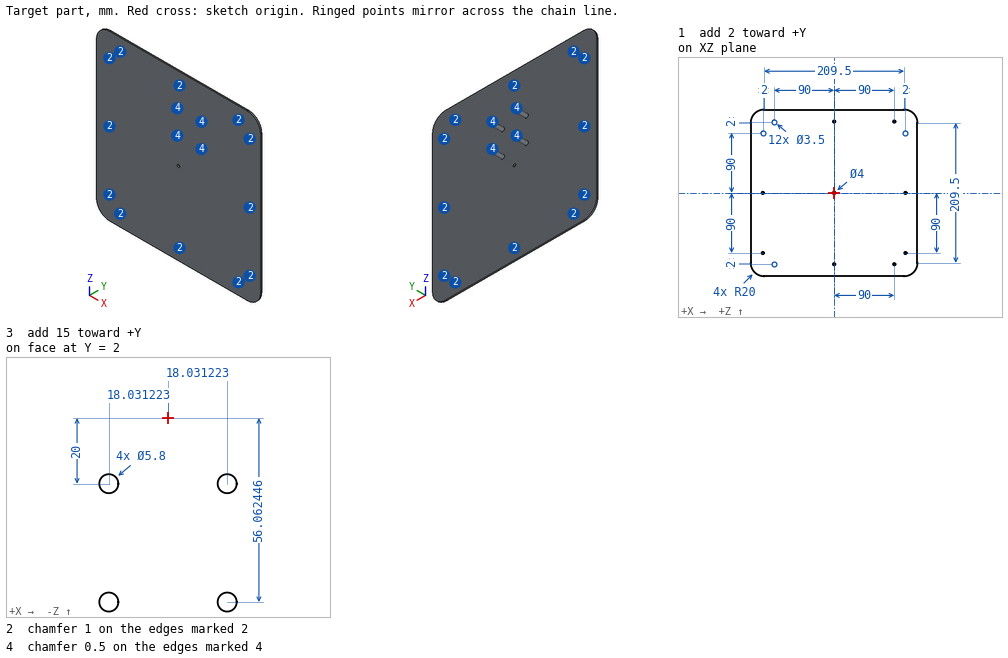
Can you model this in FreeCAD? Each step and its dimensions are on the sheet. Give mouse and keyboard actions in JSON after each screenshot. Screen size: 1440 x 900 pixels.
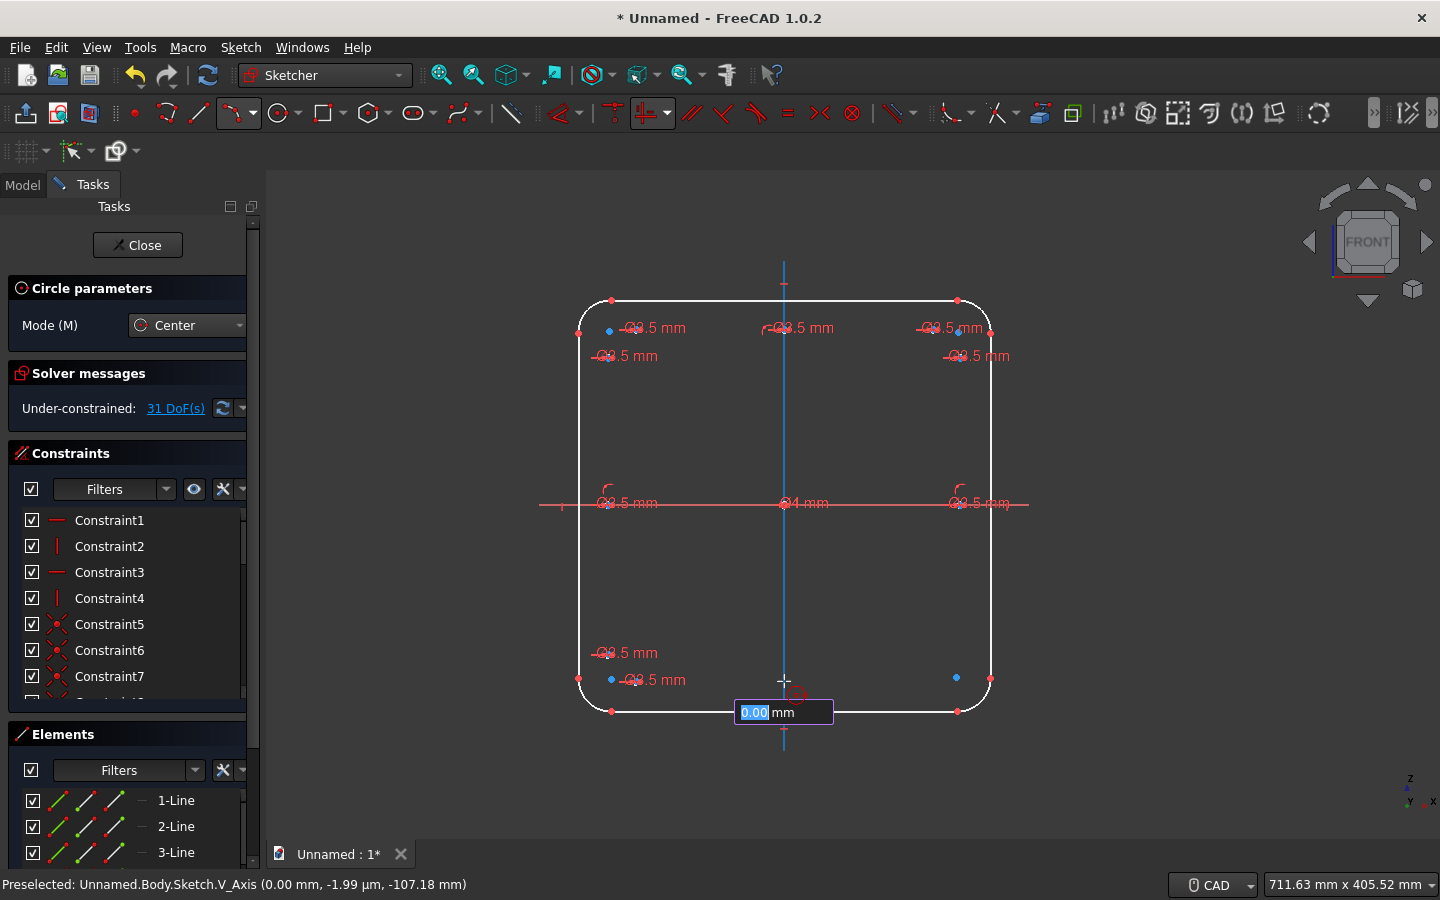
{"action": "scroll", "coordinate": [787, 680], "scroll_direction": "up", "scroll_amount": 9}
{"action": "mouse_move", "coordinate": [786, 678]}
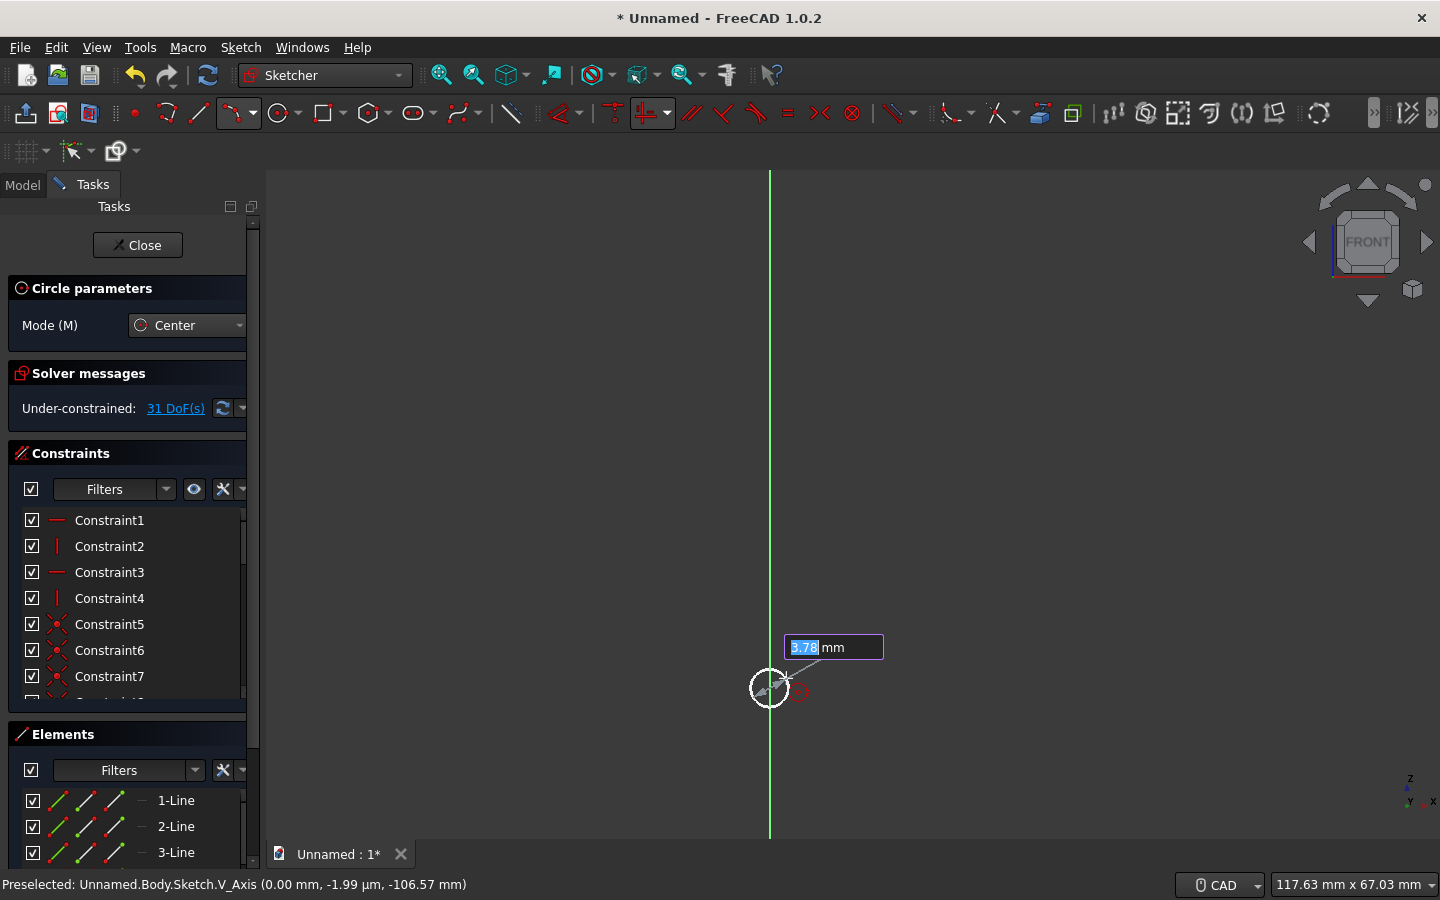
{"action": "type", "text": "3.5"}
{"action": "key", "text": "Return"}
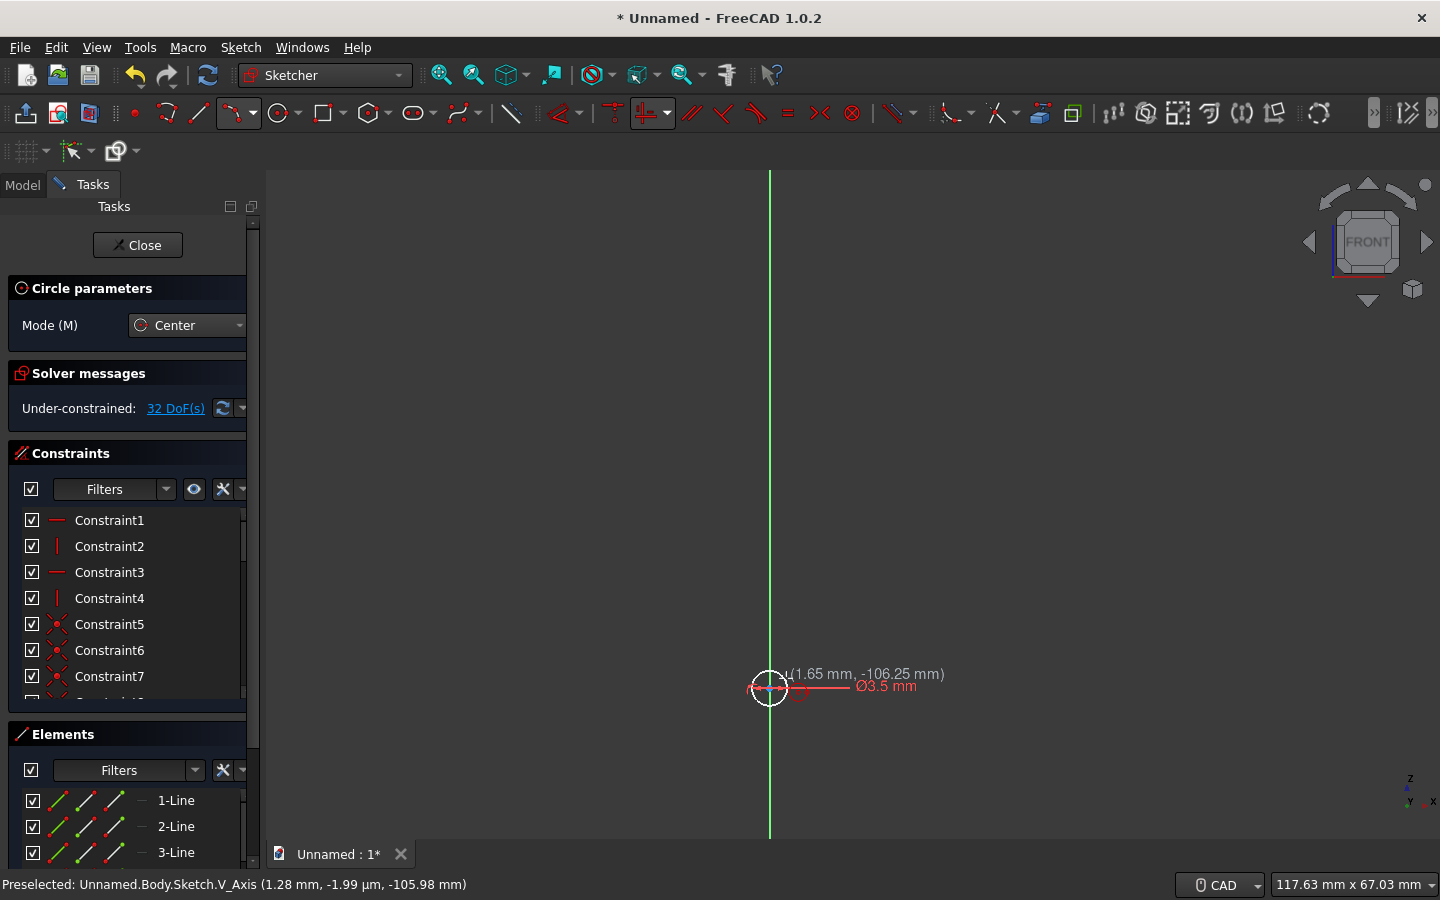
{"action": "scroll", "coordinate": [787, 680], "scroll_direction": "down", "scroll_amount": 9}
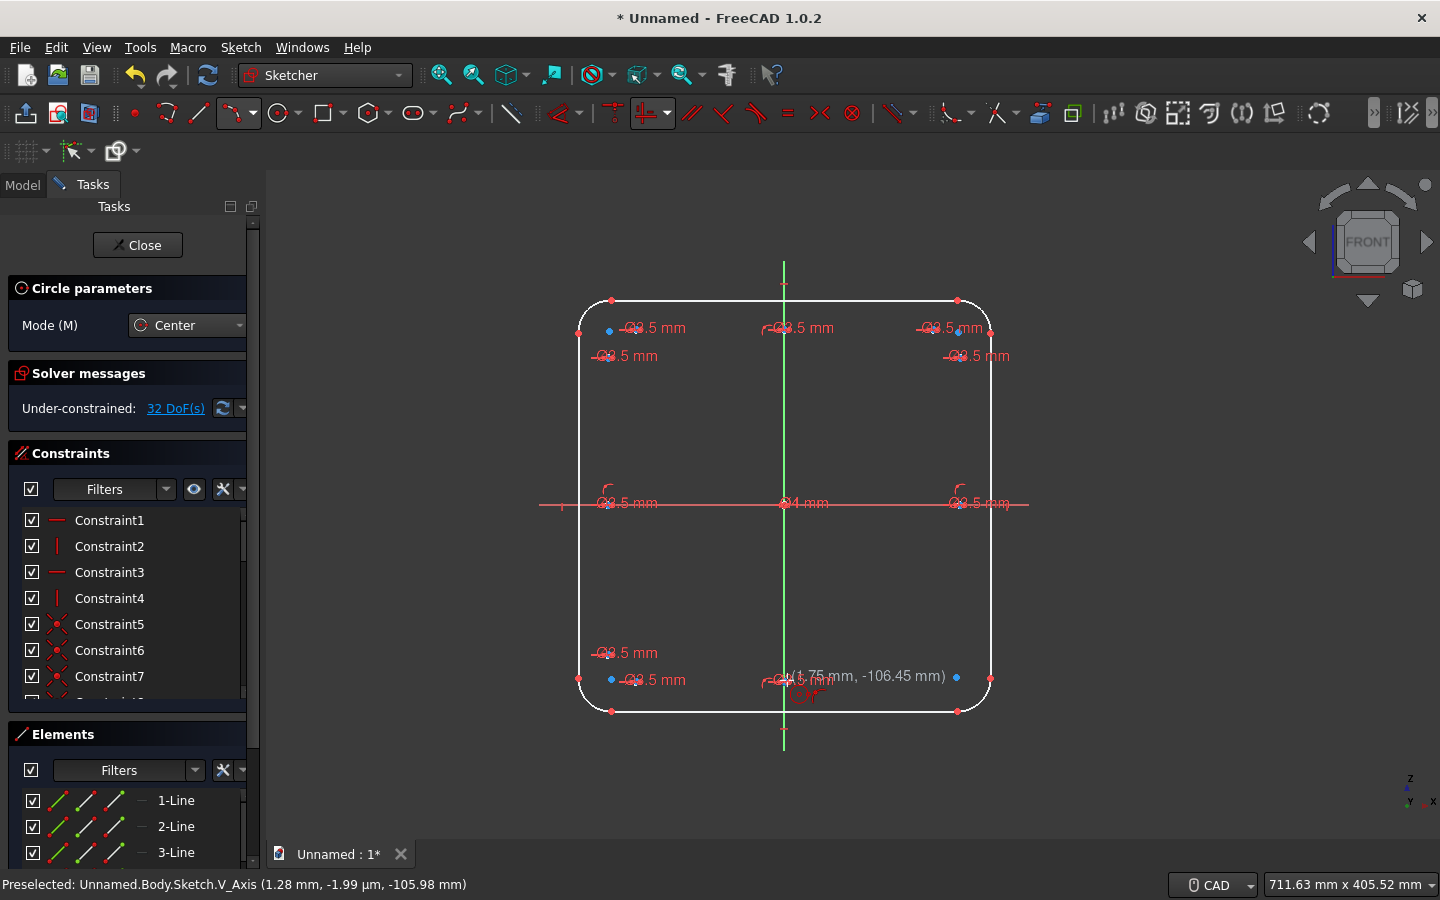
{"action": "scroll", "coordinate": [961, 654], "scroll_direction": "up", "scroll_amount": 11}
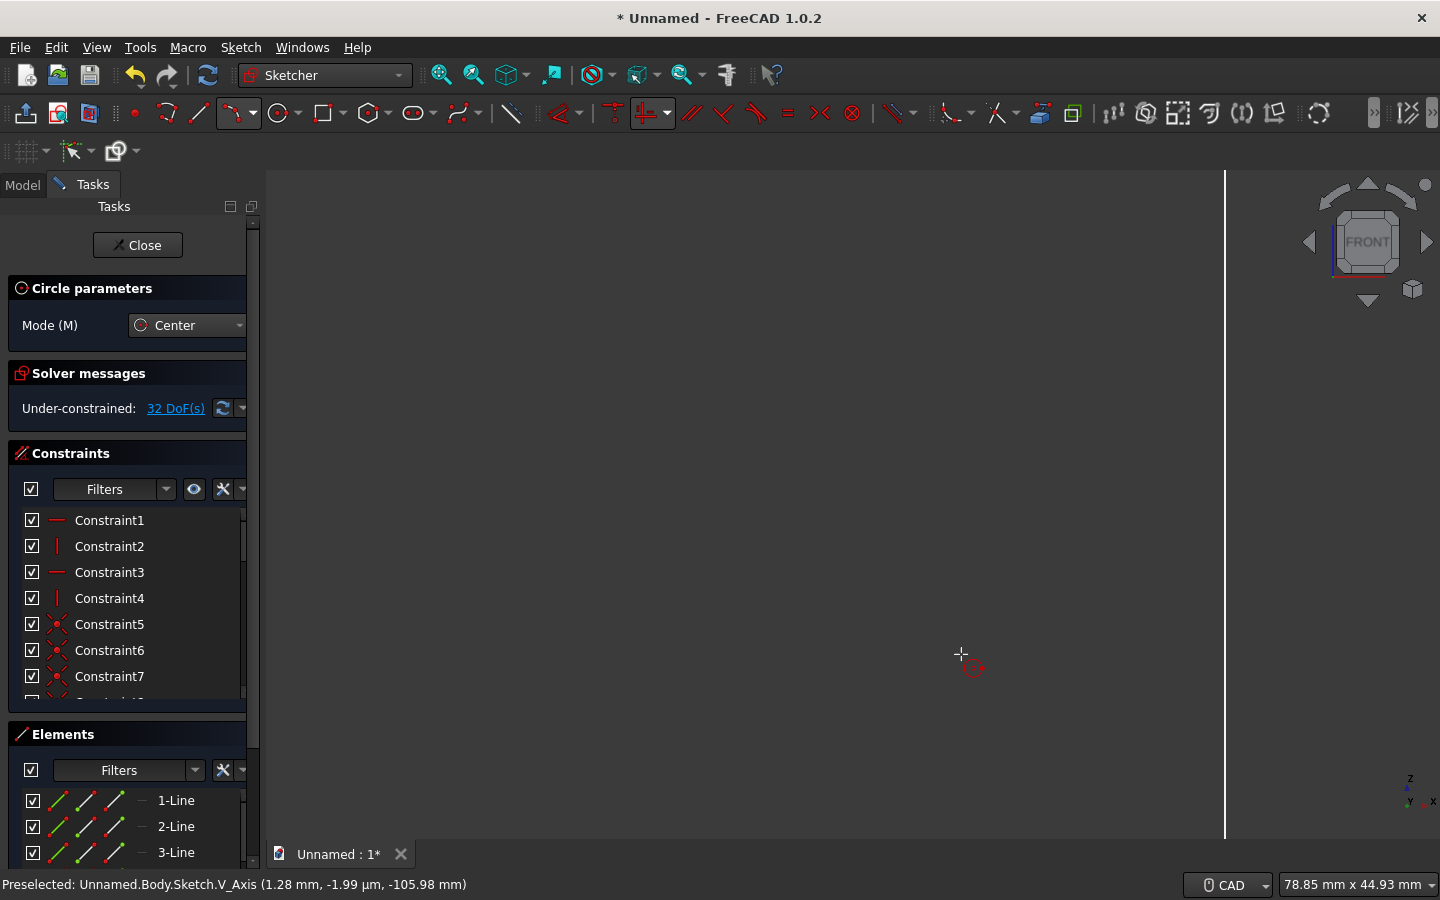
{"action": "scroll", "coordinate": [962, 654], "scroll_direction": "down", "scroll_amount": 11}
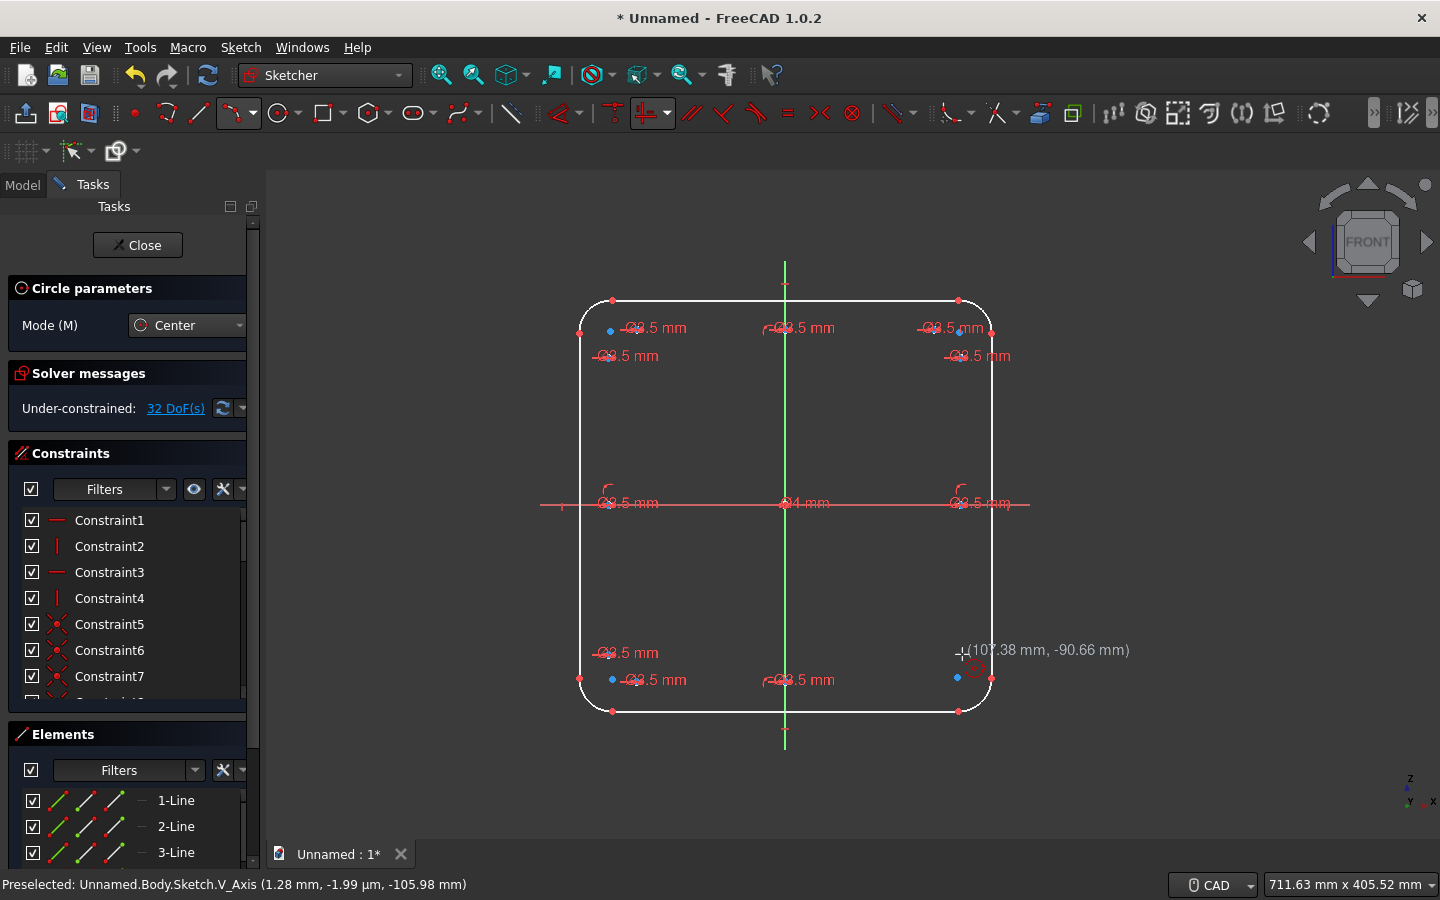
{"action": "left_click", "coordinate": [961, 654]}
{"action": "mouse_move", "coordinate": [964, 652]}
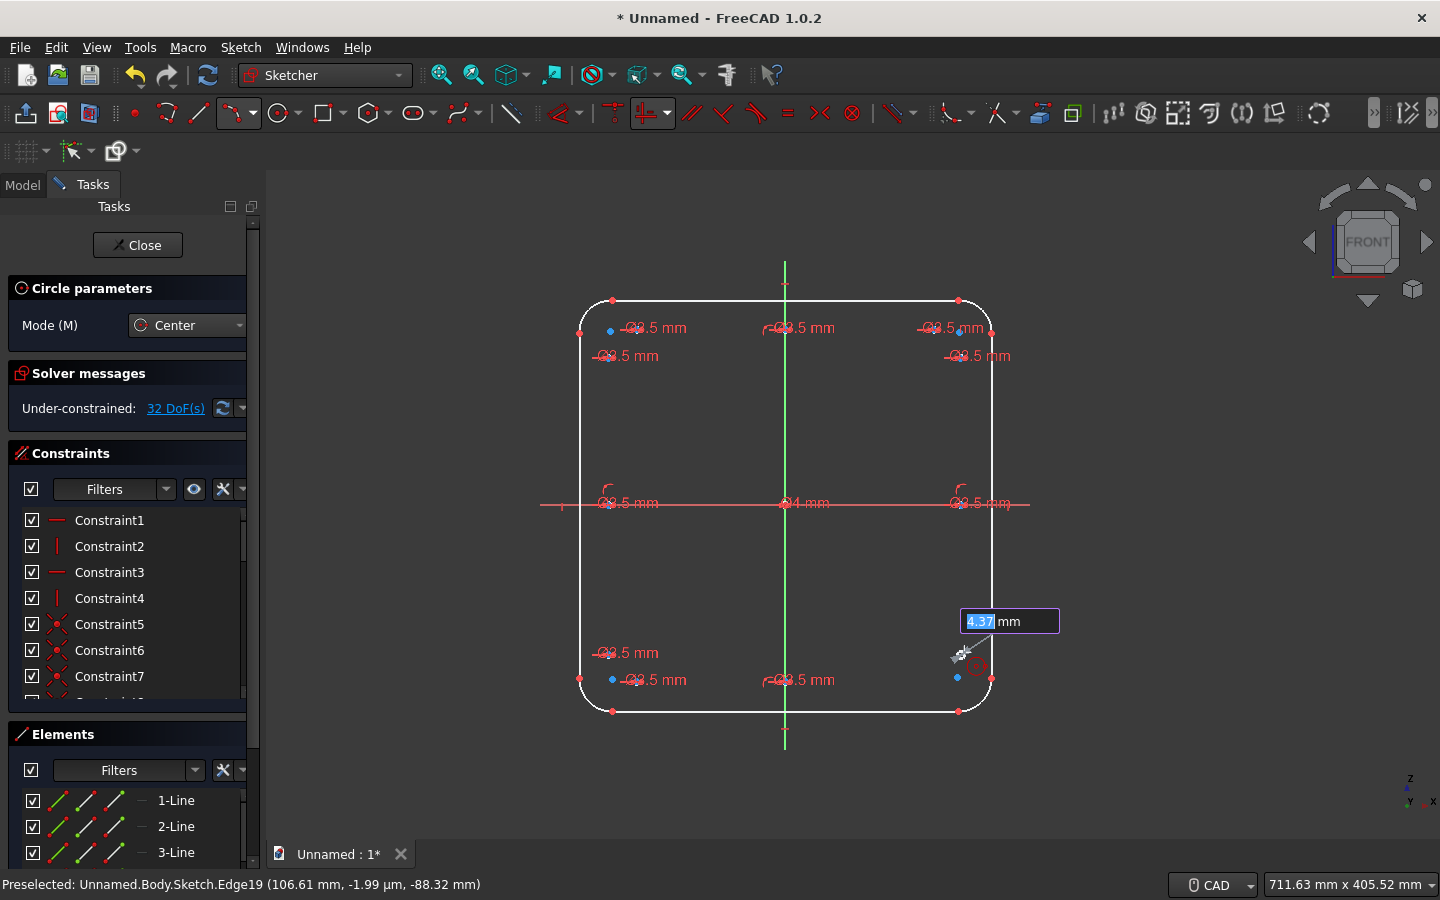
{"action": "type", "text": "3.5"}
{"action": "key", "text": "Return"}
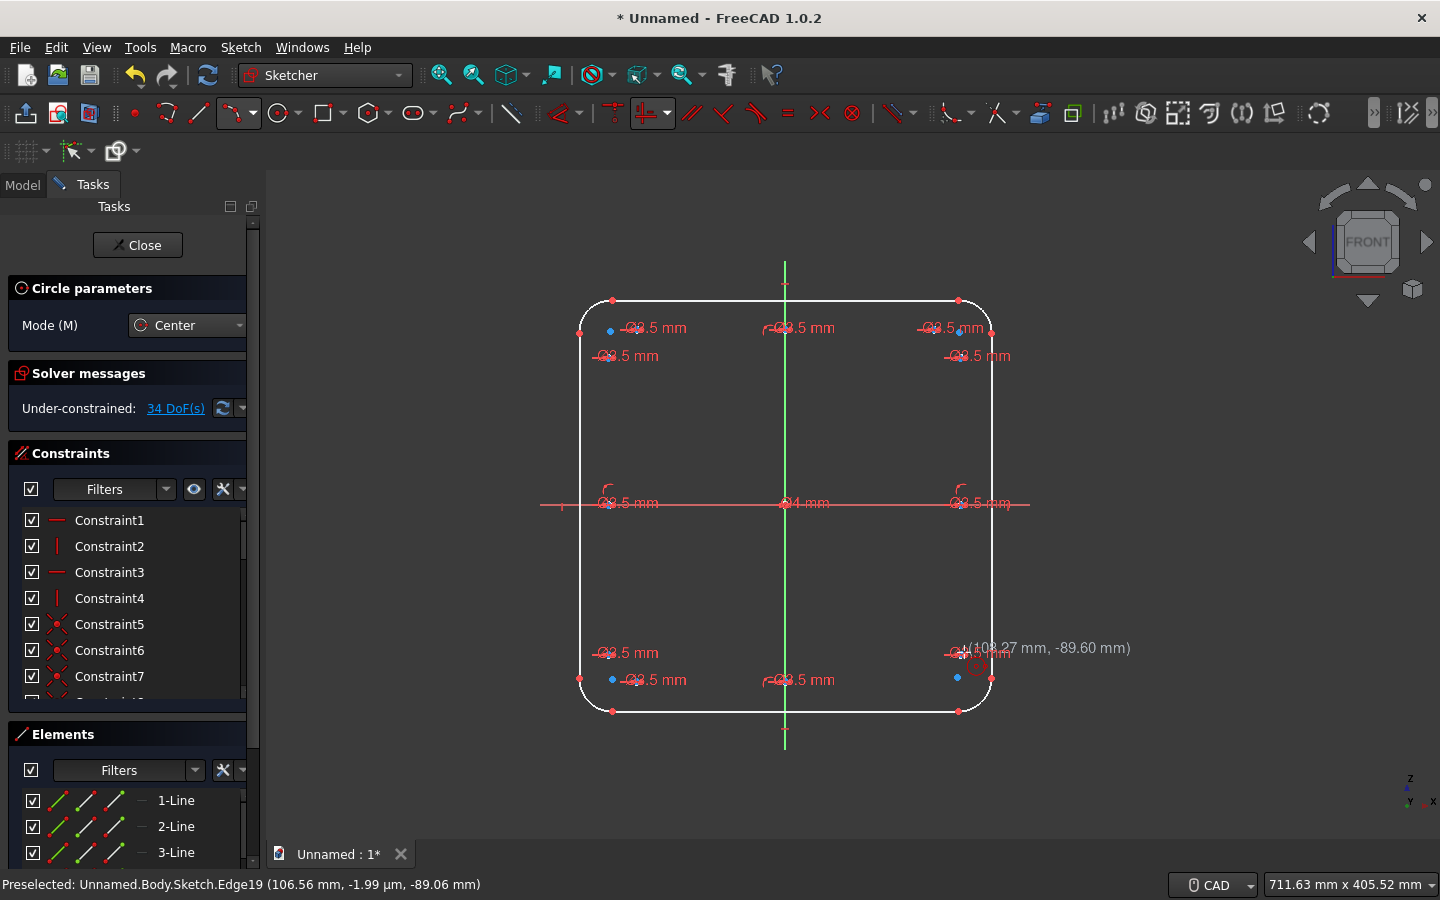
{"action": "scroll", "coordinate": [934, 681], "scroll_direction": "up", "scroll_amount": 11}